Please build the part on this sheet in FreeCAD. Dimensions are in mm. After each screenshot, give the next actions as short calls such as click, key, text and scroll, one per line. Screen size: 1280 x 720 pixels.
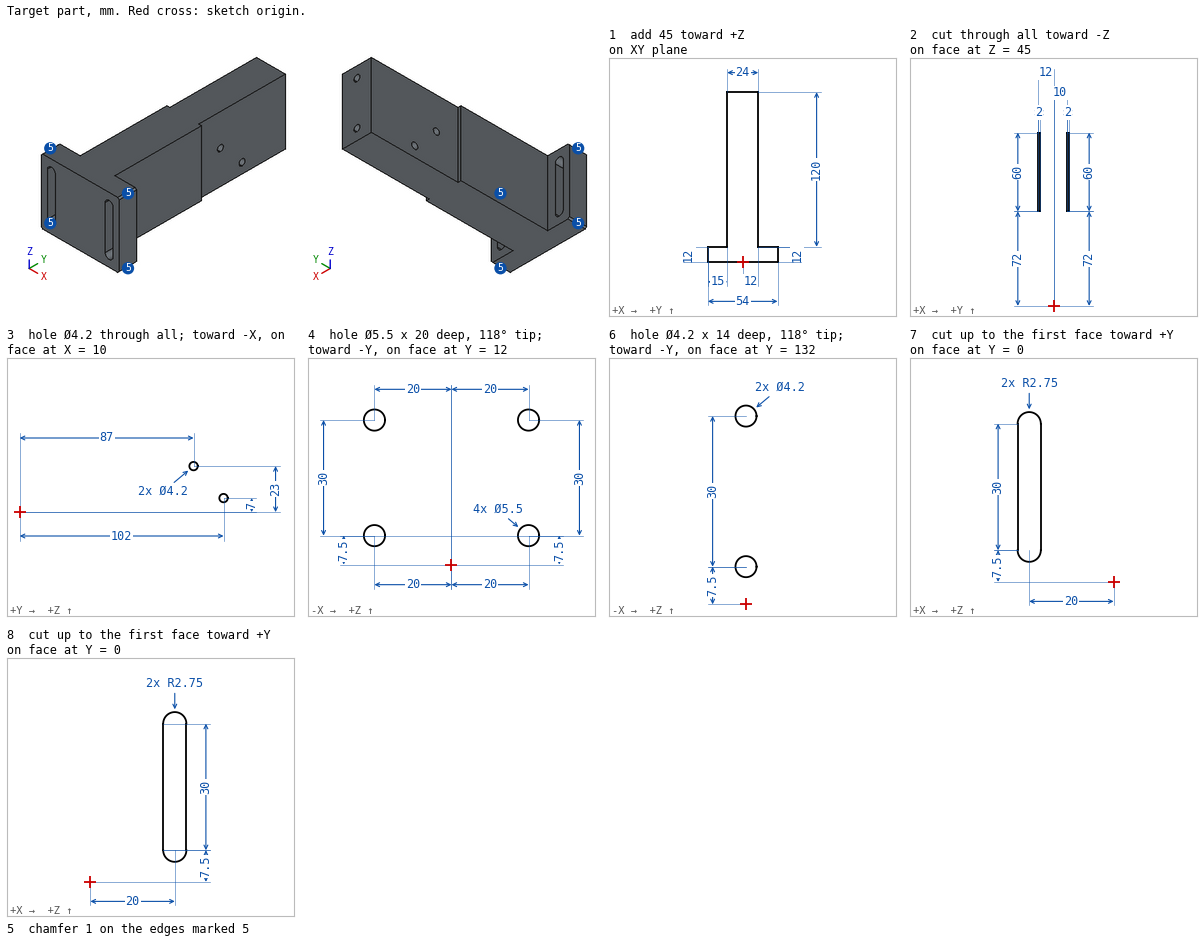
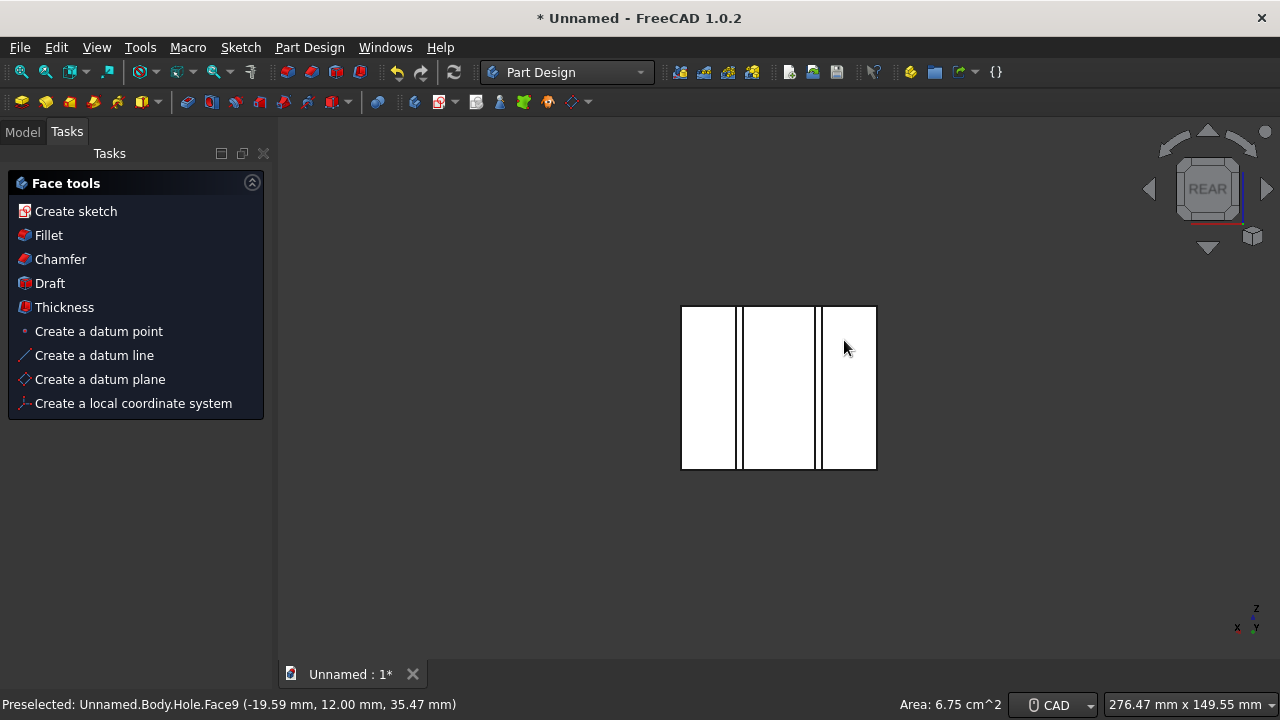
click(440, 102)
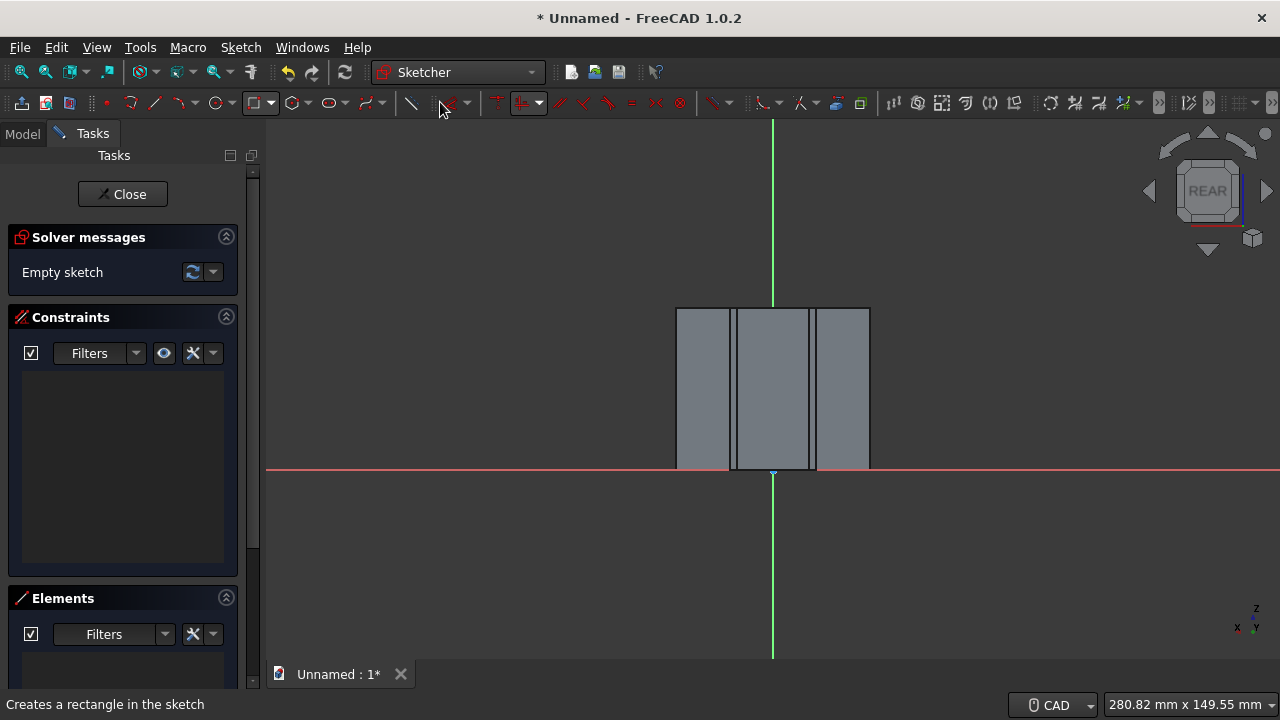
scroll(829, 405, up, 4)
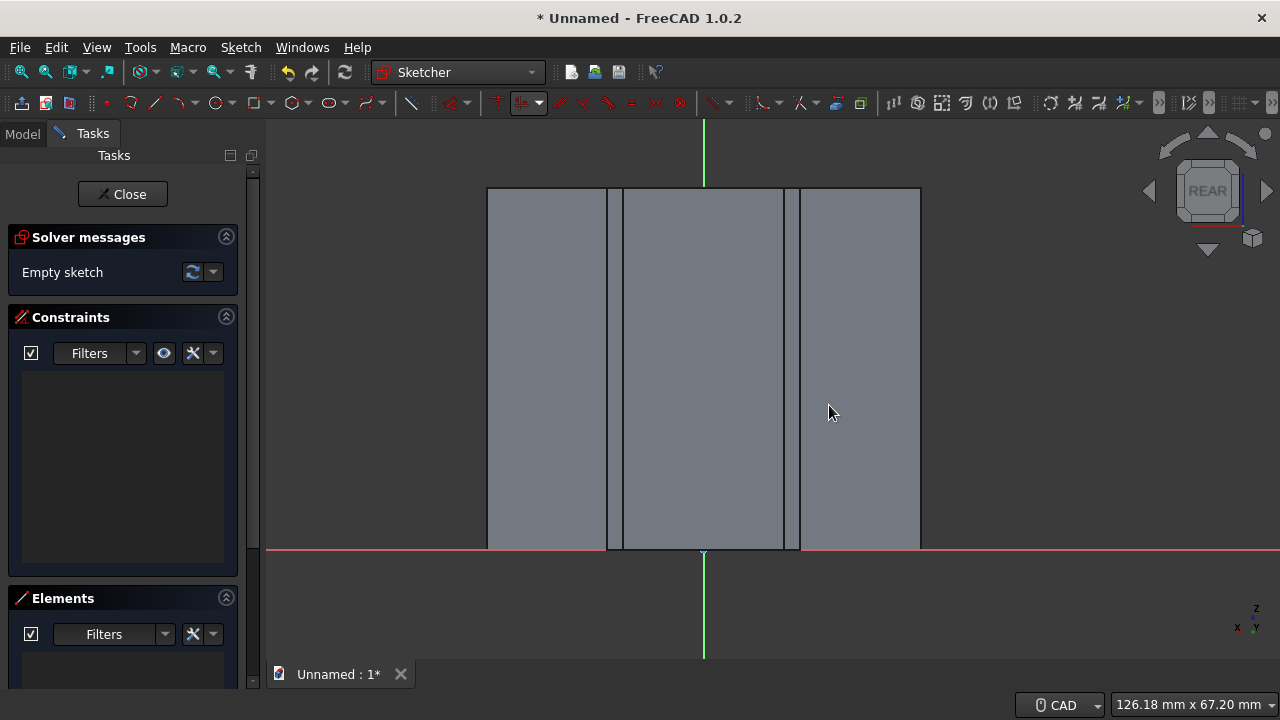
click(216, 104)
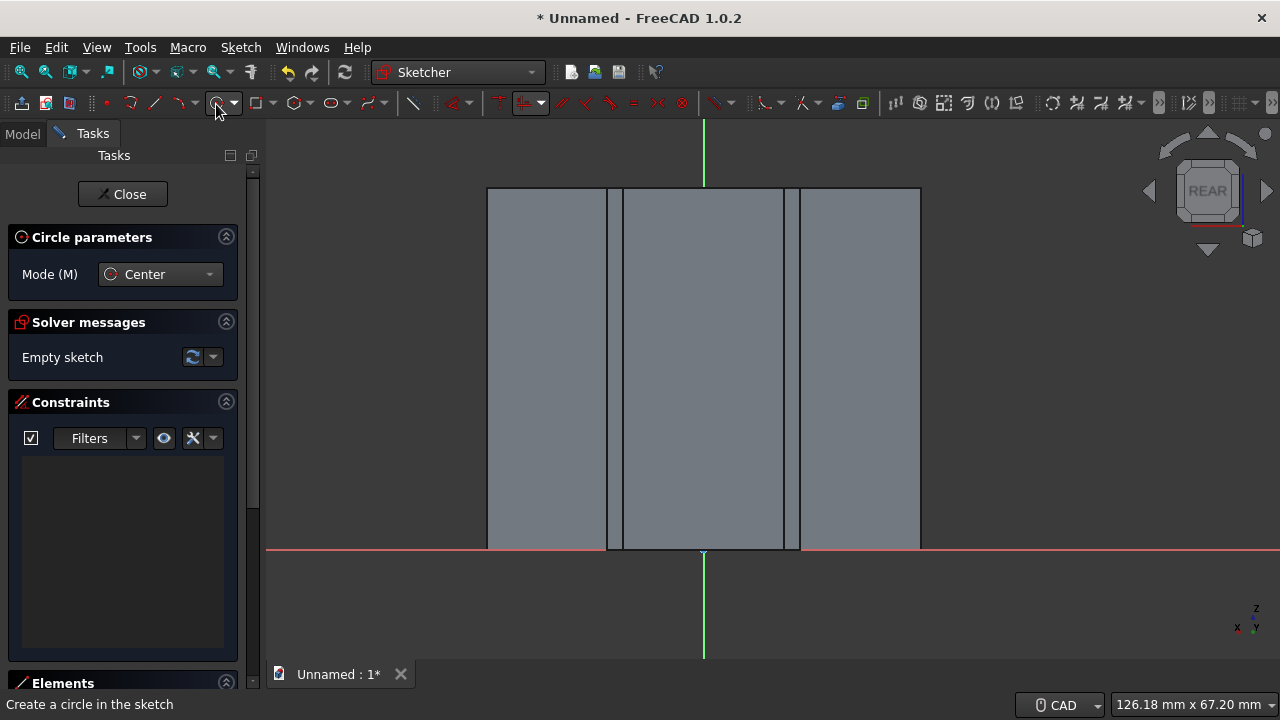
click(864, 489)
move(880, 474)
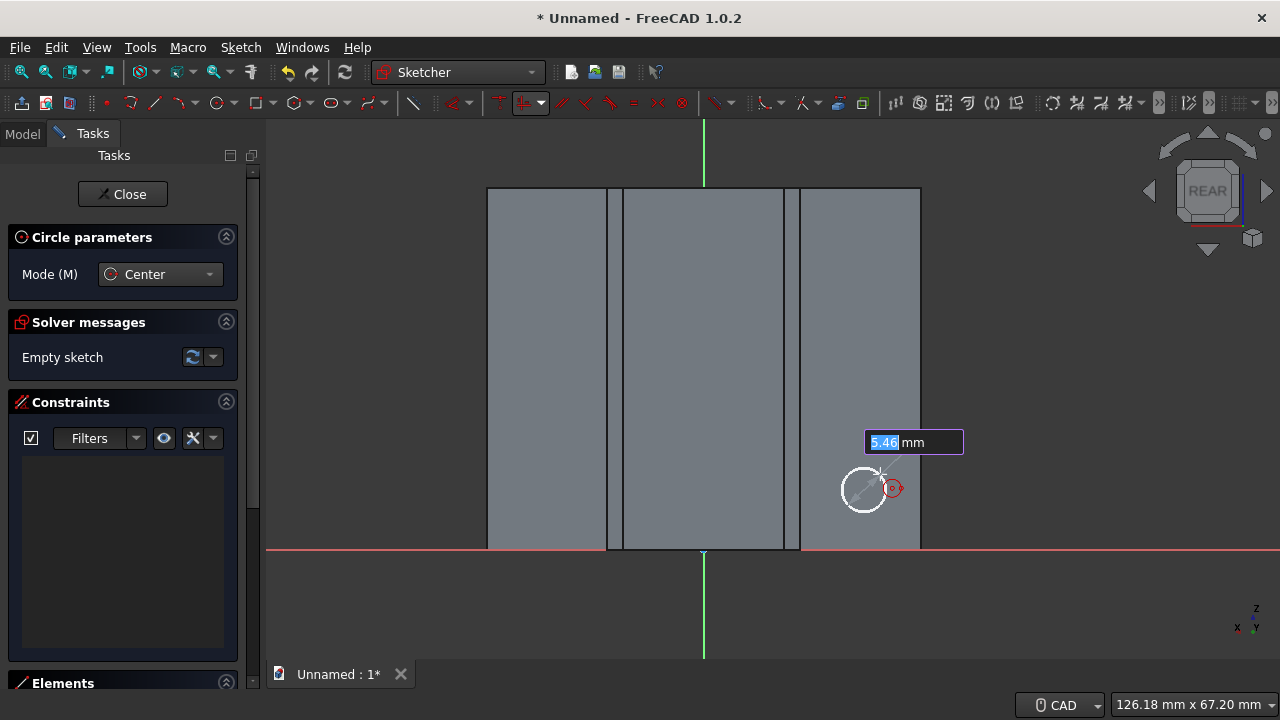
text(5.5)
key(Return)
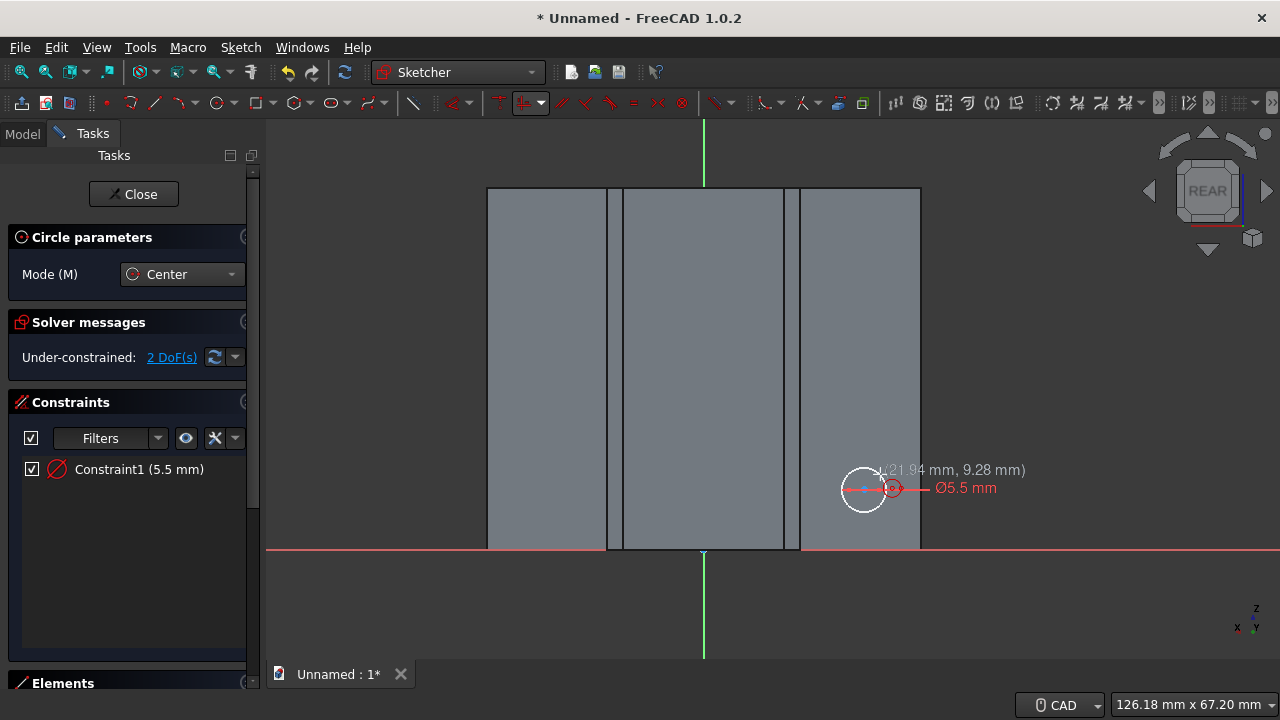
click(864, 248)
move(880, 233)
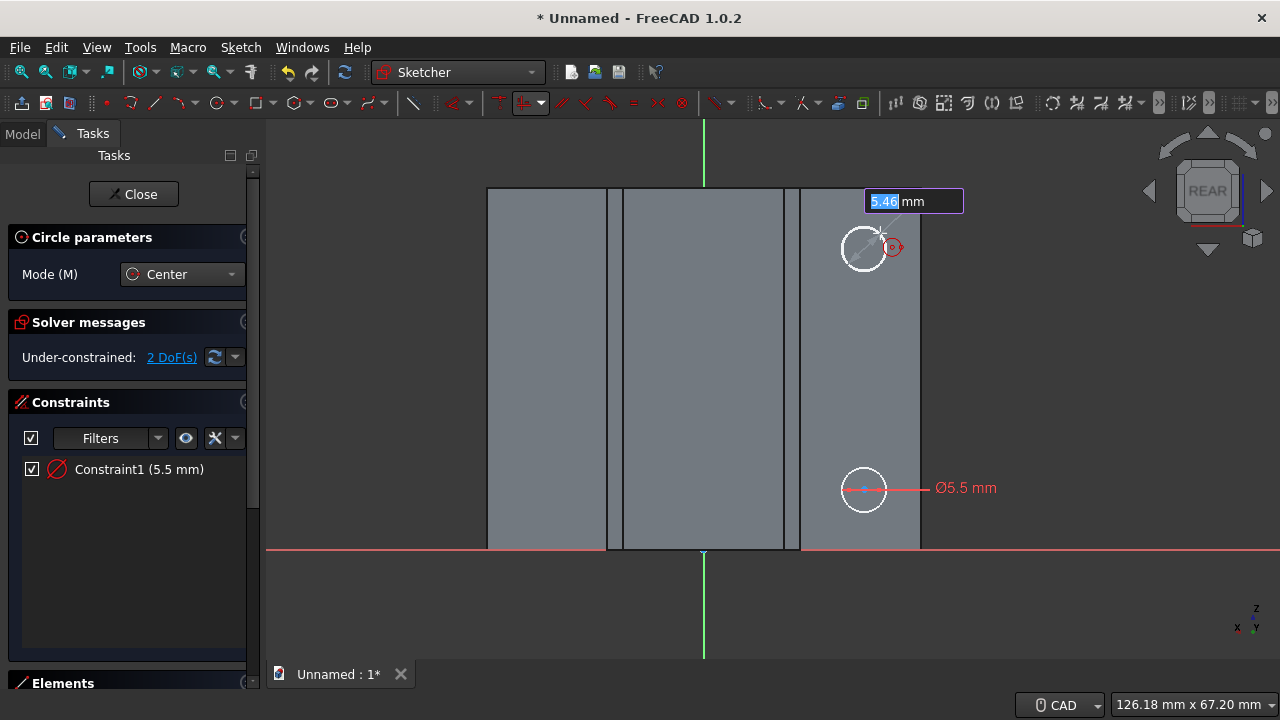
text(5.5)
key(Return)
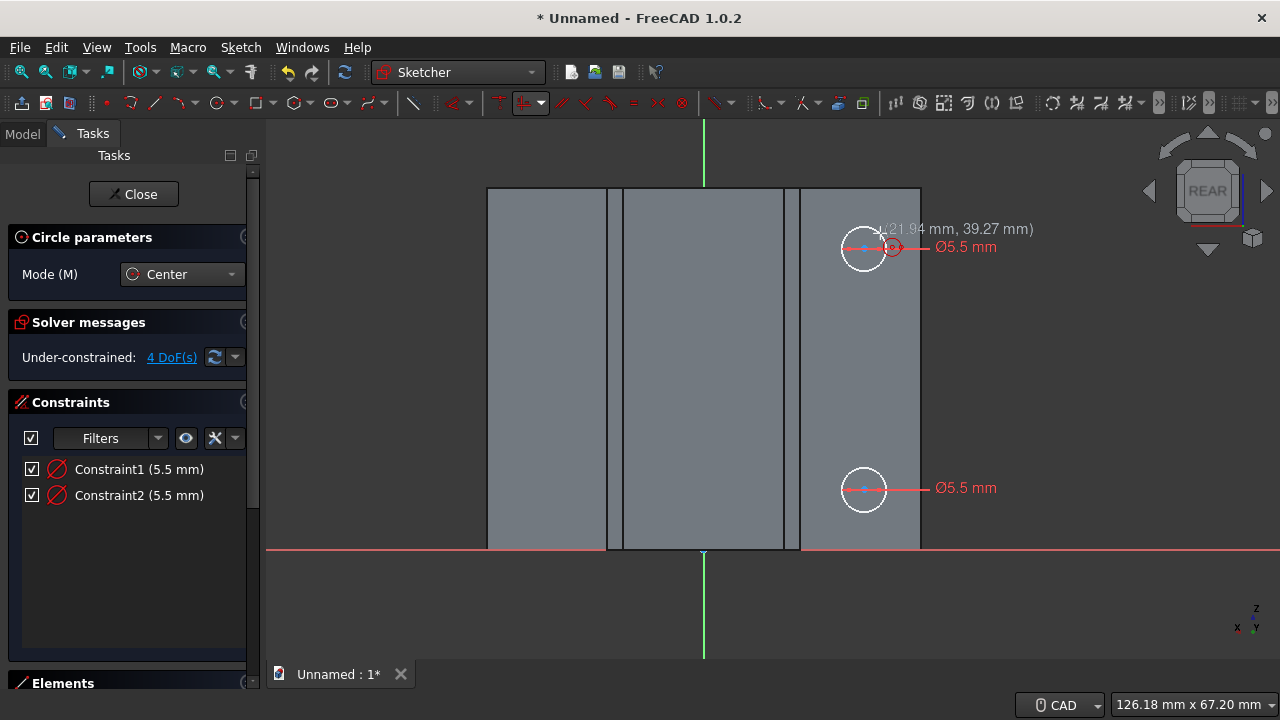
click(543, 248)
move(559, 233)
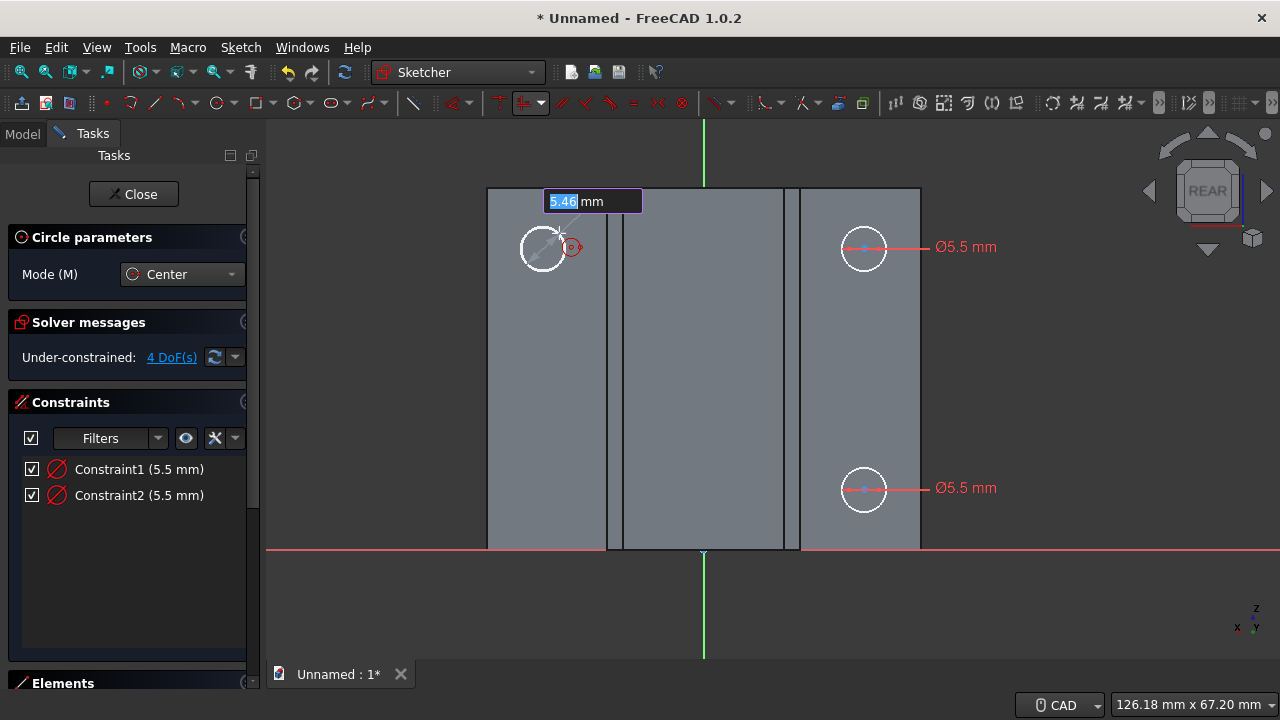
text(5.5)
key(Return)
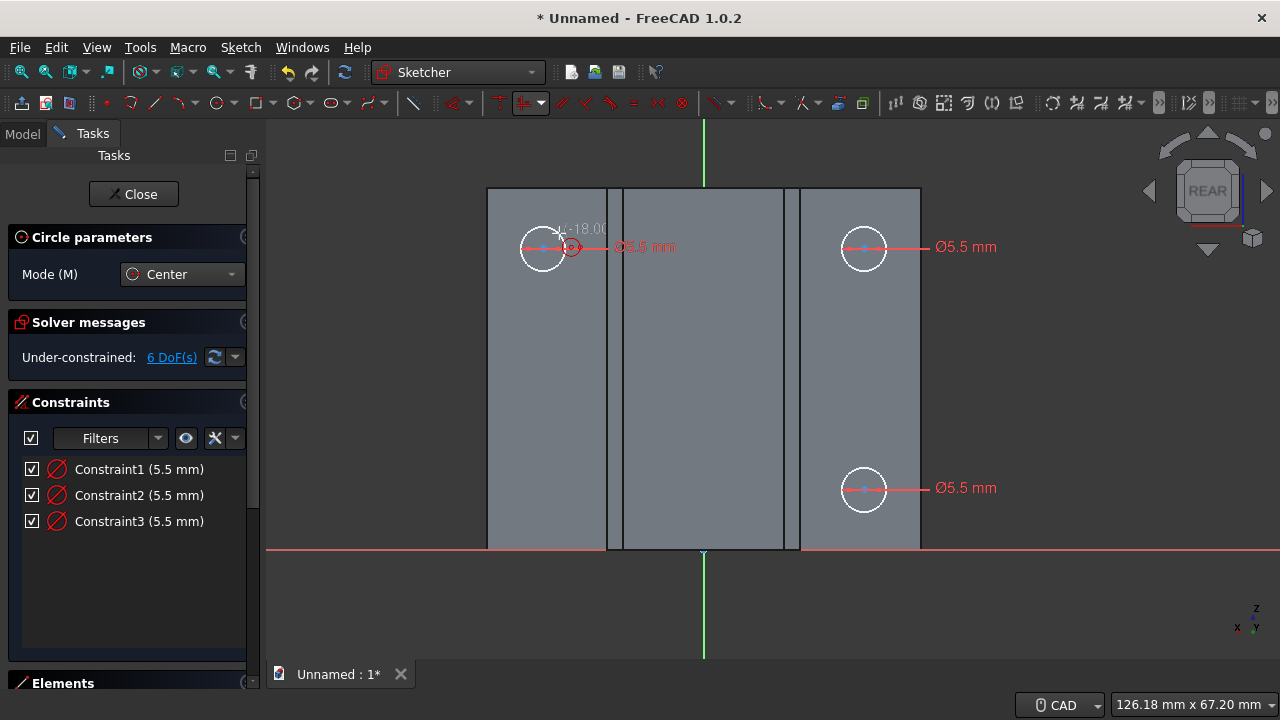
click(543, 489)
move(559, 474)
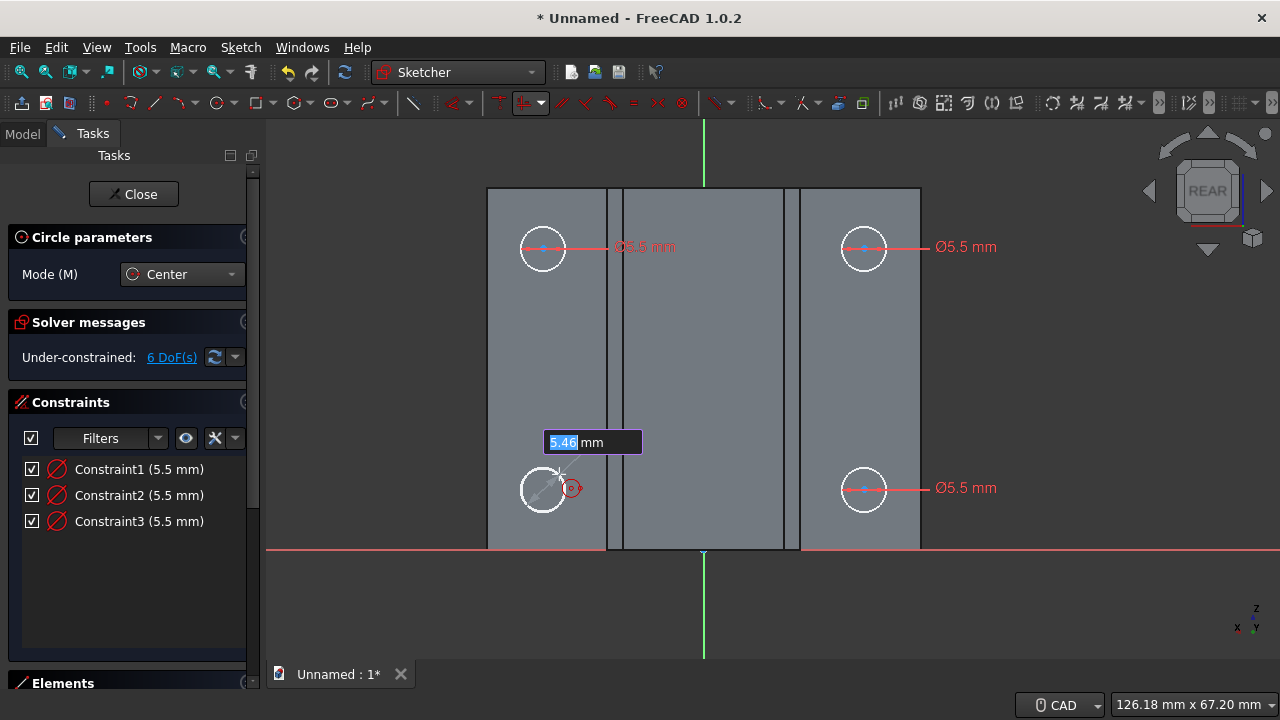
text(5.5)
key(Return)
key(Escape)